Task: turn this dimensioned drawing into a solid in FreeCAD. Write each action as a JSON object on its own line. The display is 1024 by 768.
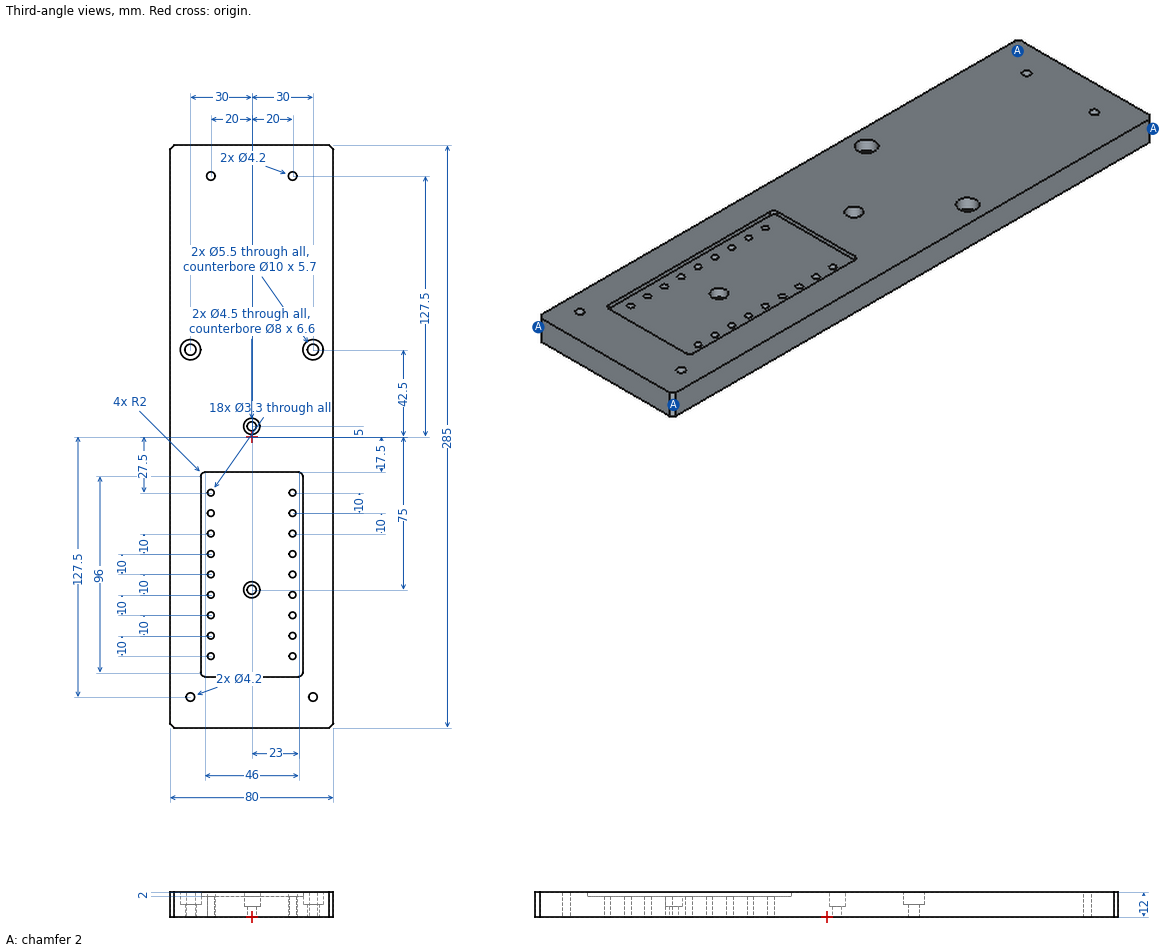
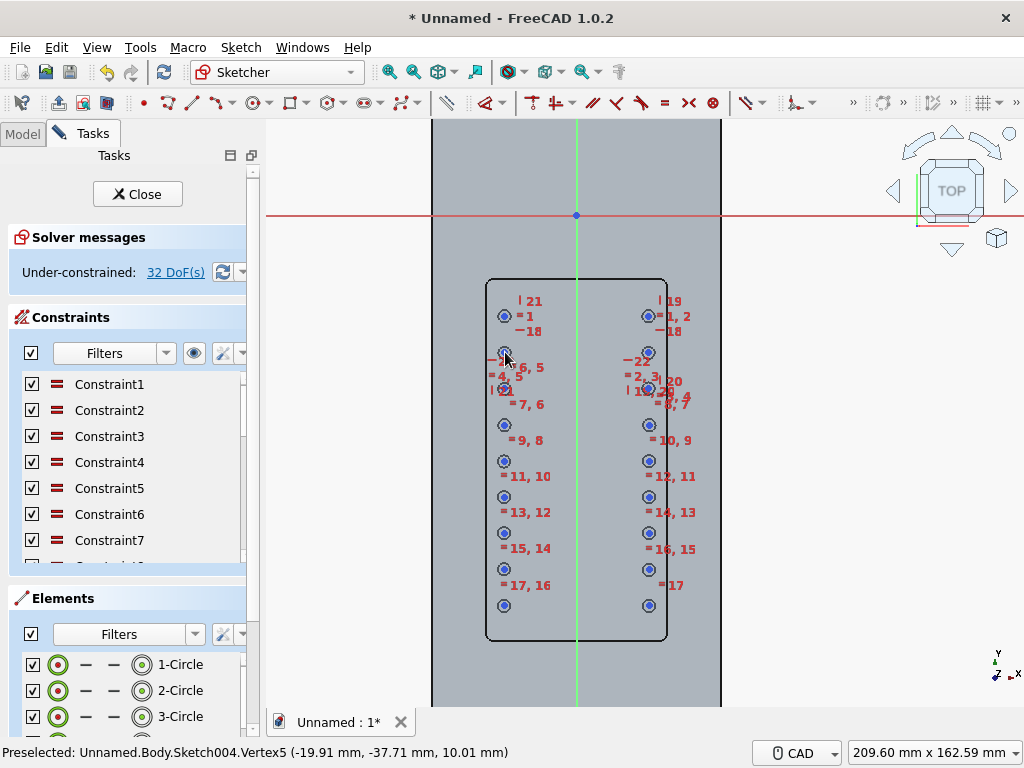
{"action": "left_click", "coordinate": [503, 351]}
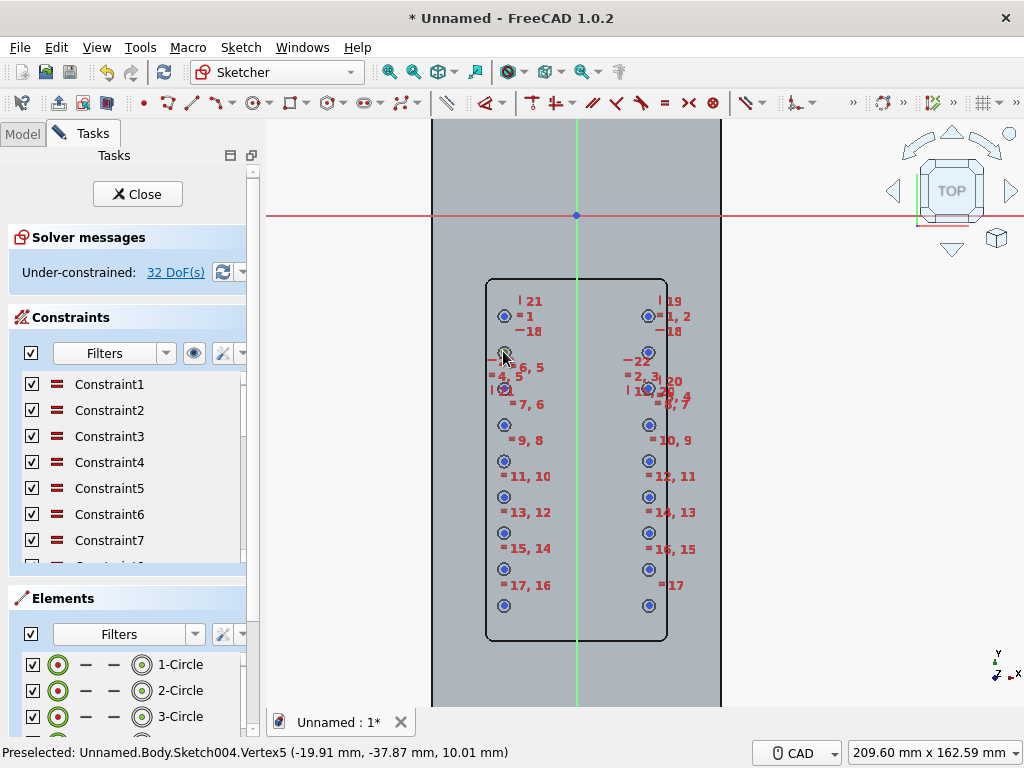
{"action": "scroll", "coordinate": [504, 389], "scroll_direction": "up", "scroll_amount": 4}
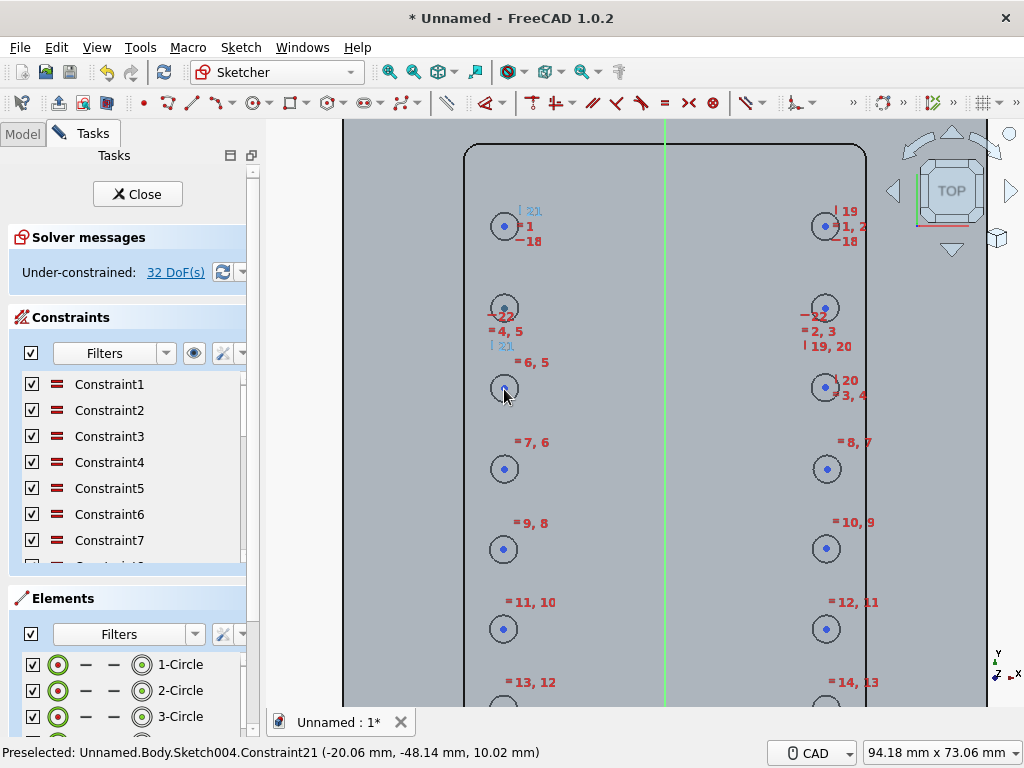
{"action": "left_click", "coordinate": [505, 388]}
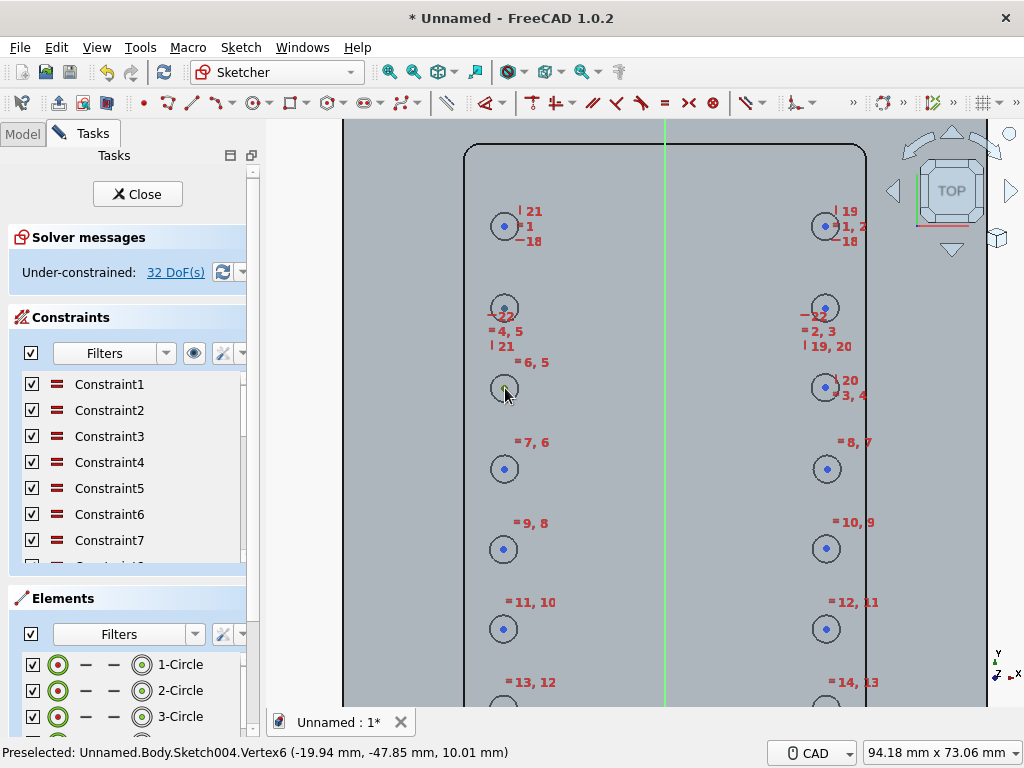
{"action": "key", "text": "v"}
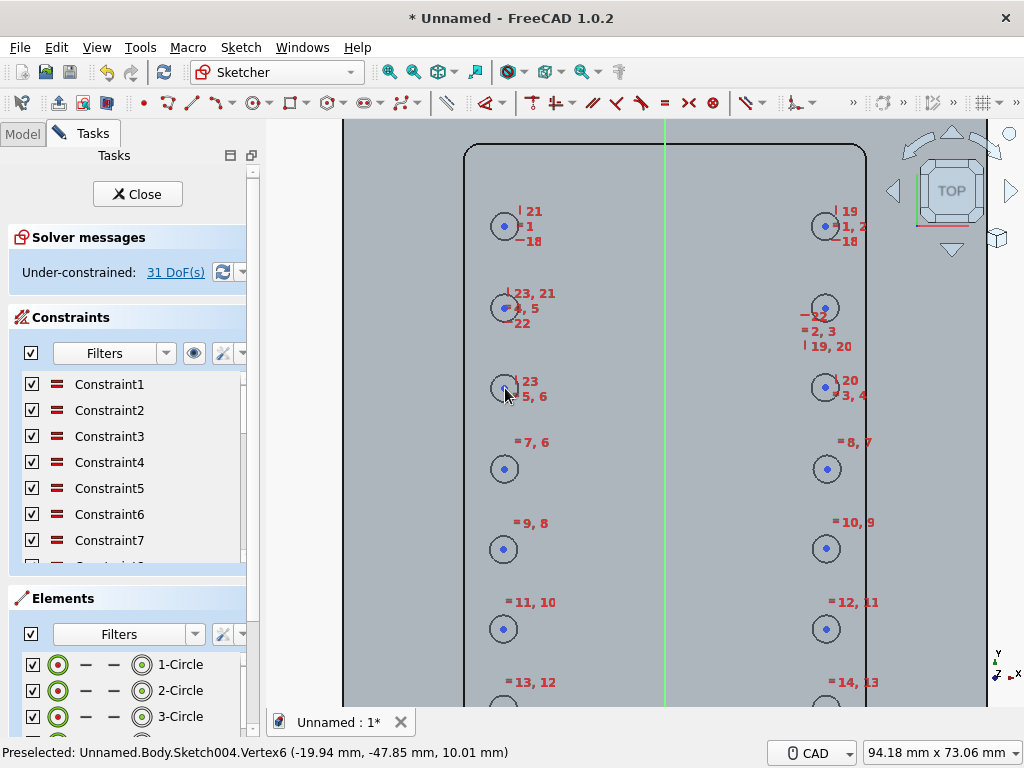
{"action": "left_click", "coordinate": [825, 388]}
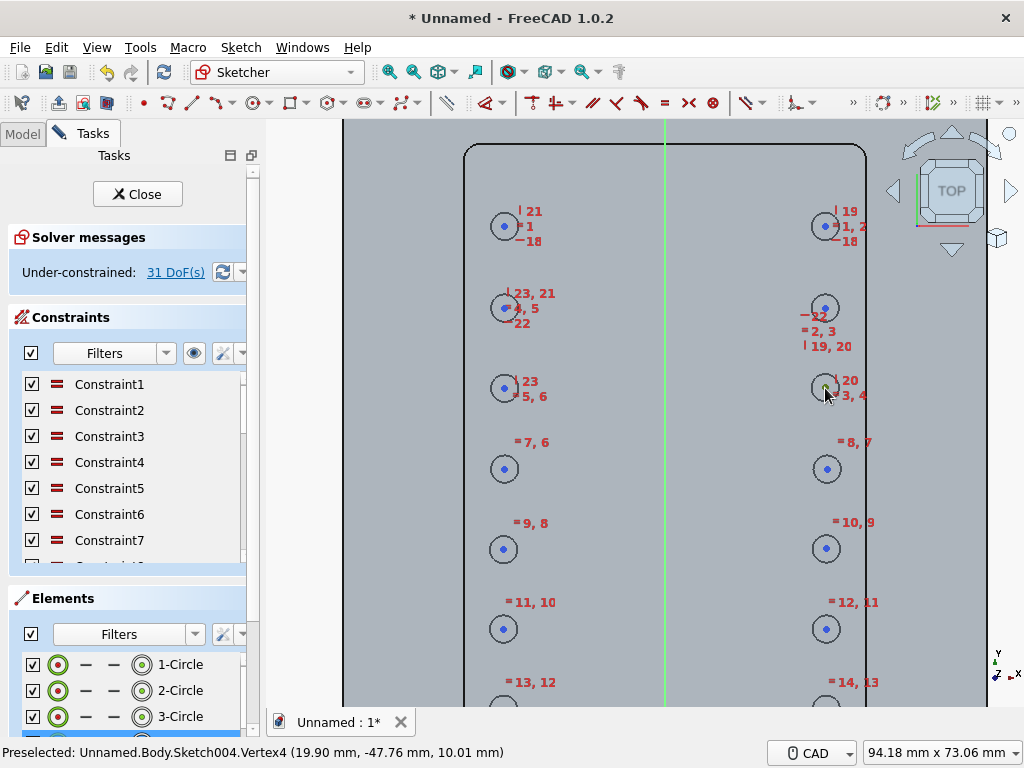
{"action": "left_click", "coordinate": [505, 388]}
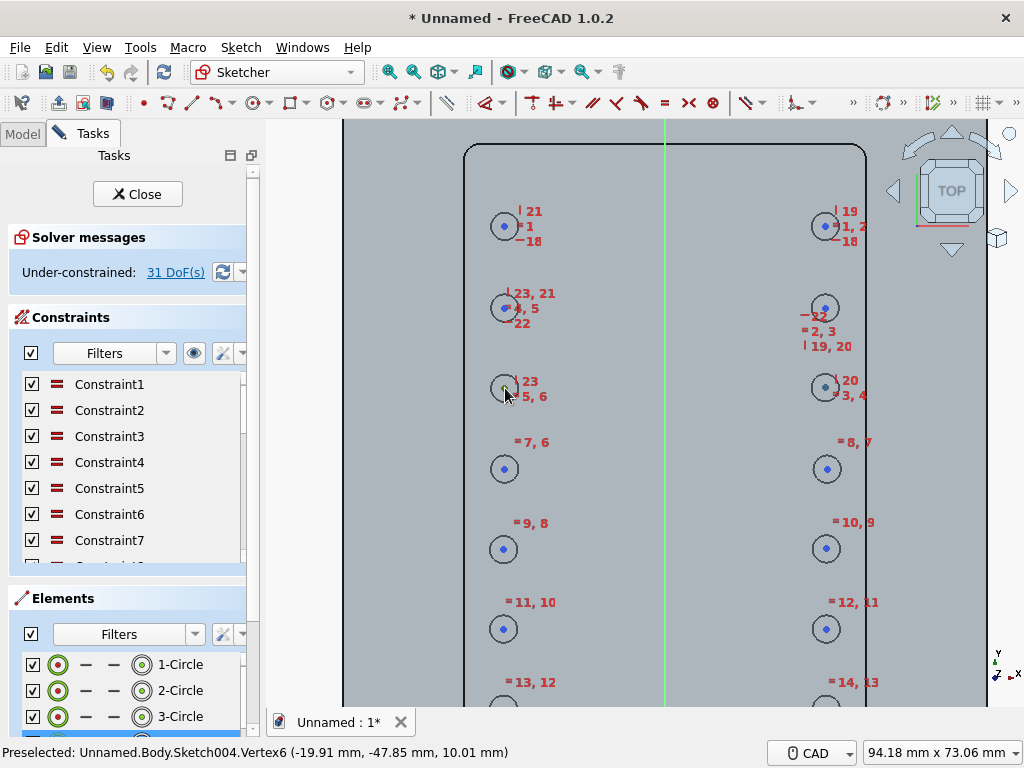
{"action": "key", "text": "h"}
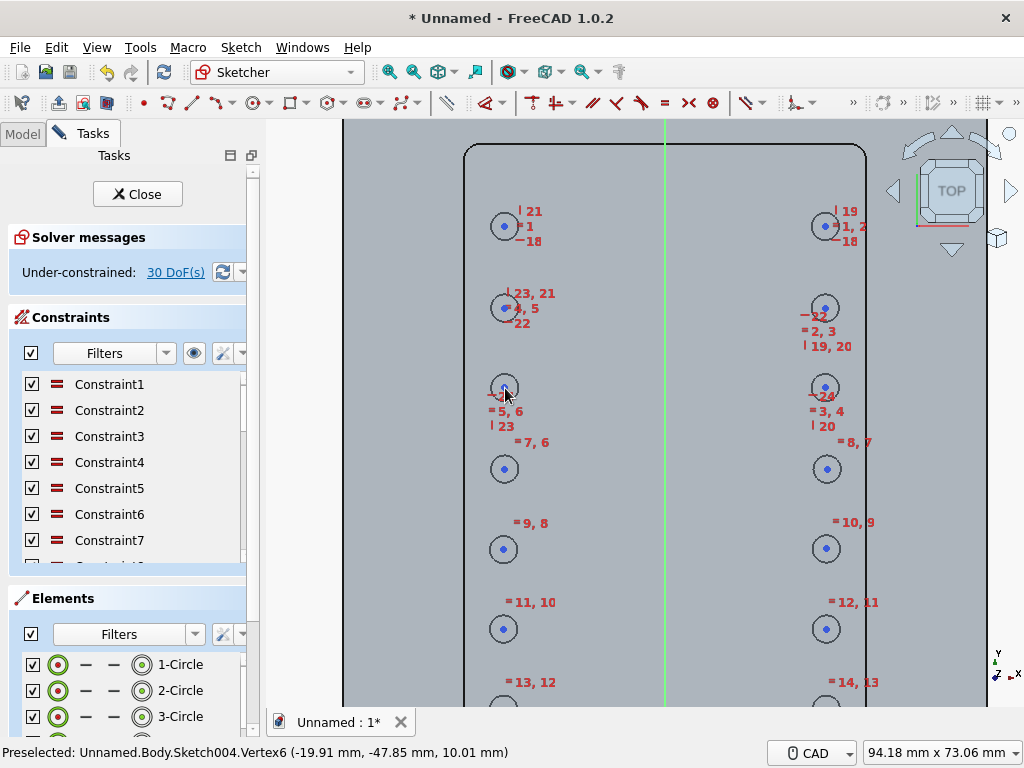
{"action": "left_click", "coordinate": [503, 386]}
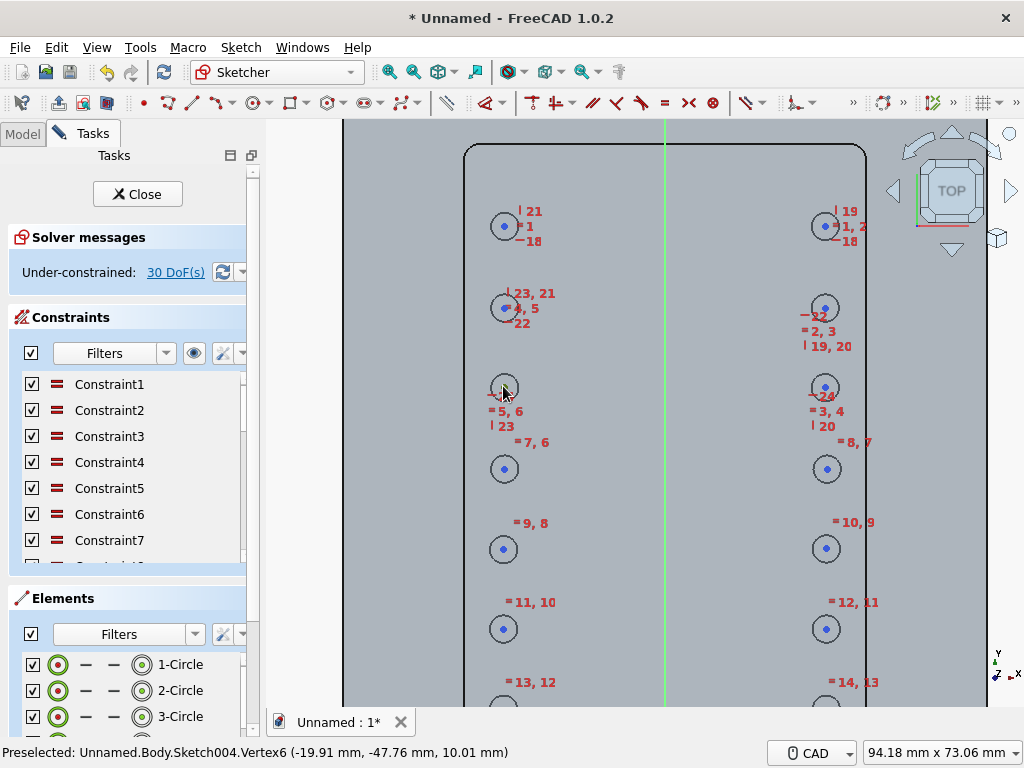
{"action": "left_click", "coordinate": [505, 469]}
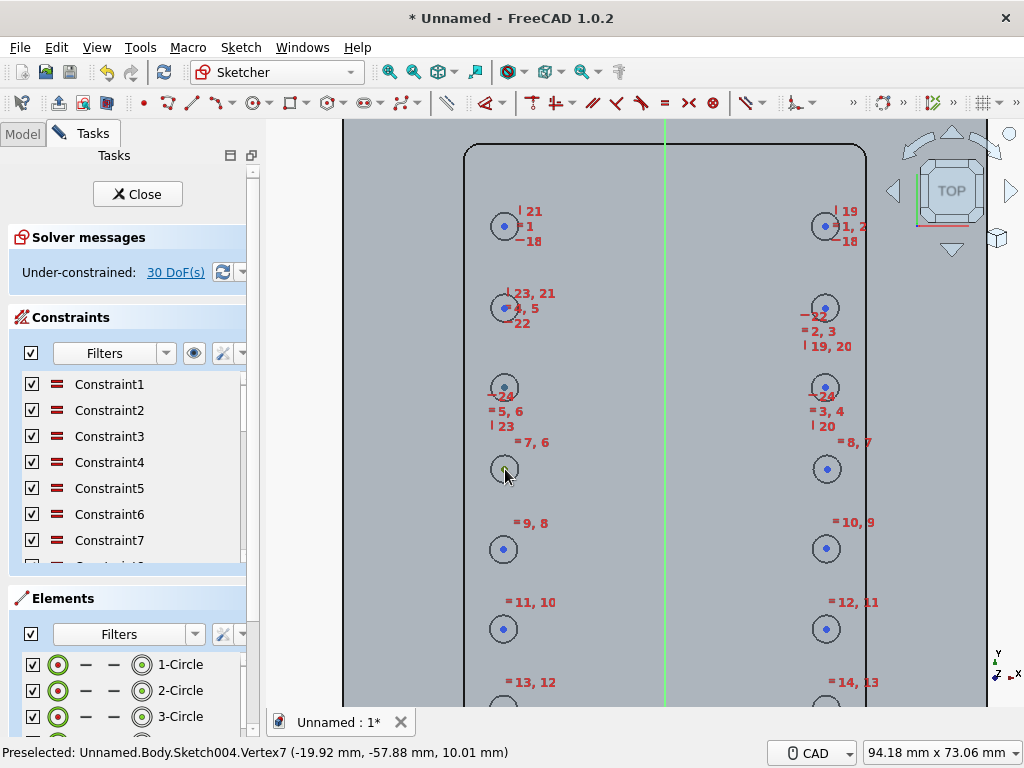
{"action": "left_click", "coordinate": [574, 104]}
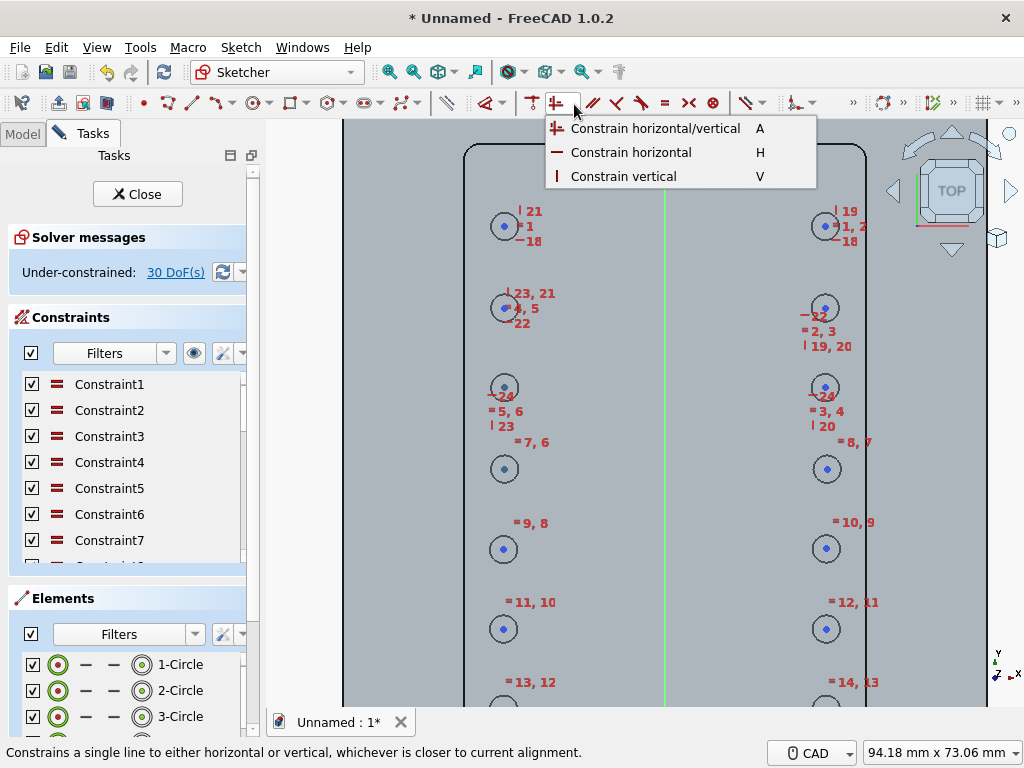
{"action": "left_click", "coordinate": [681, 176]}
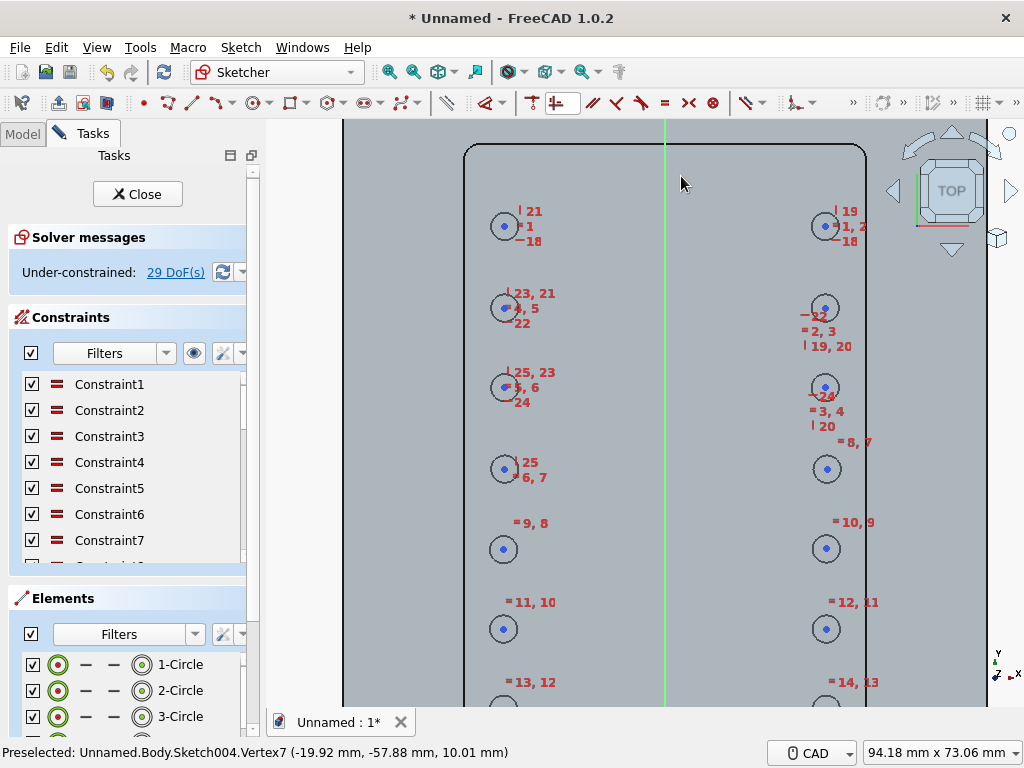
{"action": "left_click", "coordinate": [825, 388]}